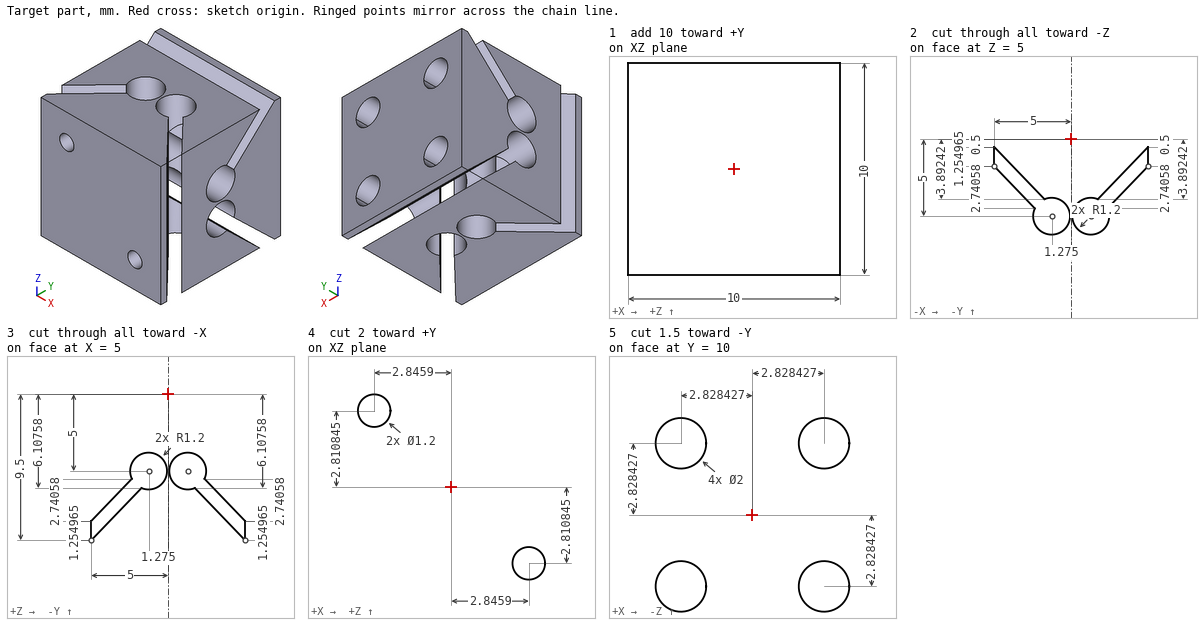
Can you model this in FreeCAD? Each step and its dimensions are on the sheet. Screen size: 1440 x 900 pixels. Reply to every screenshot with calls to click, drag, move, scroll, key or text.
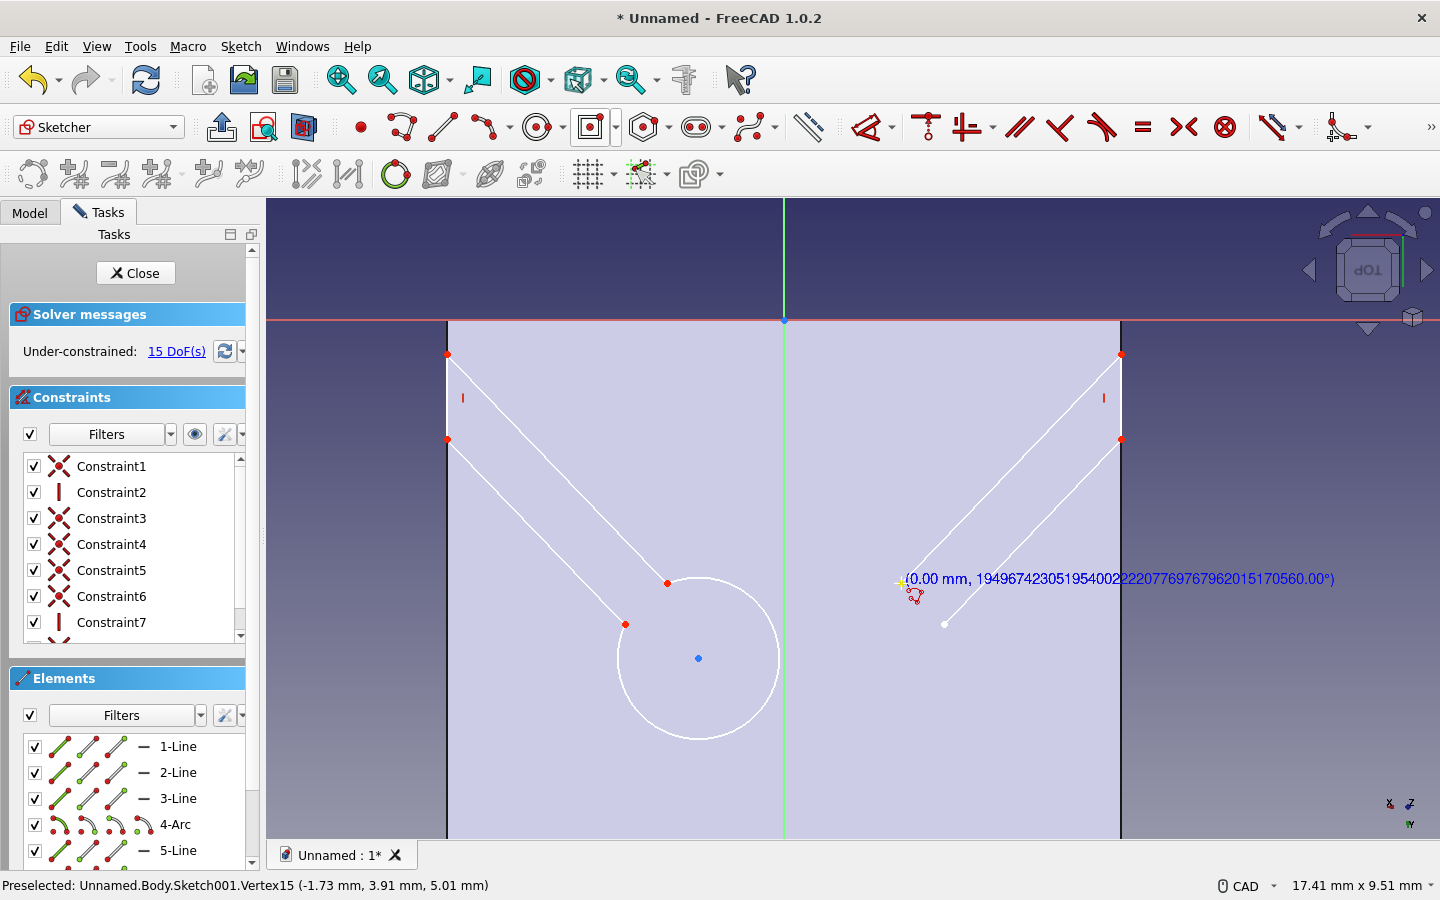
click(484, 128)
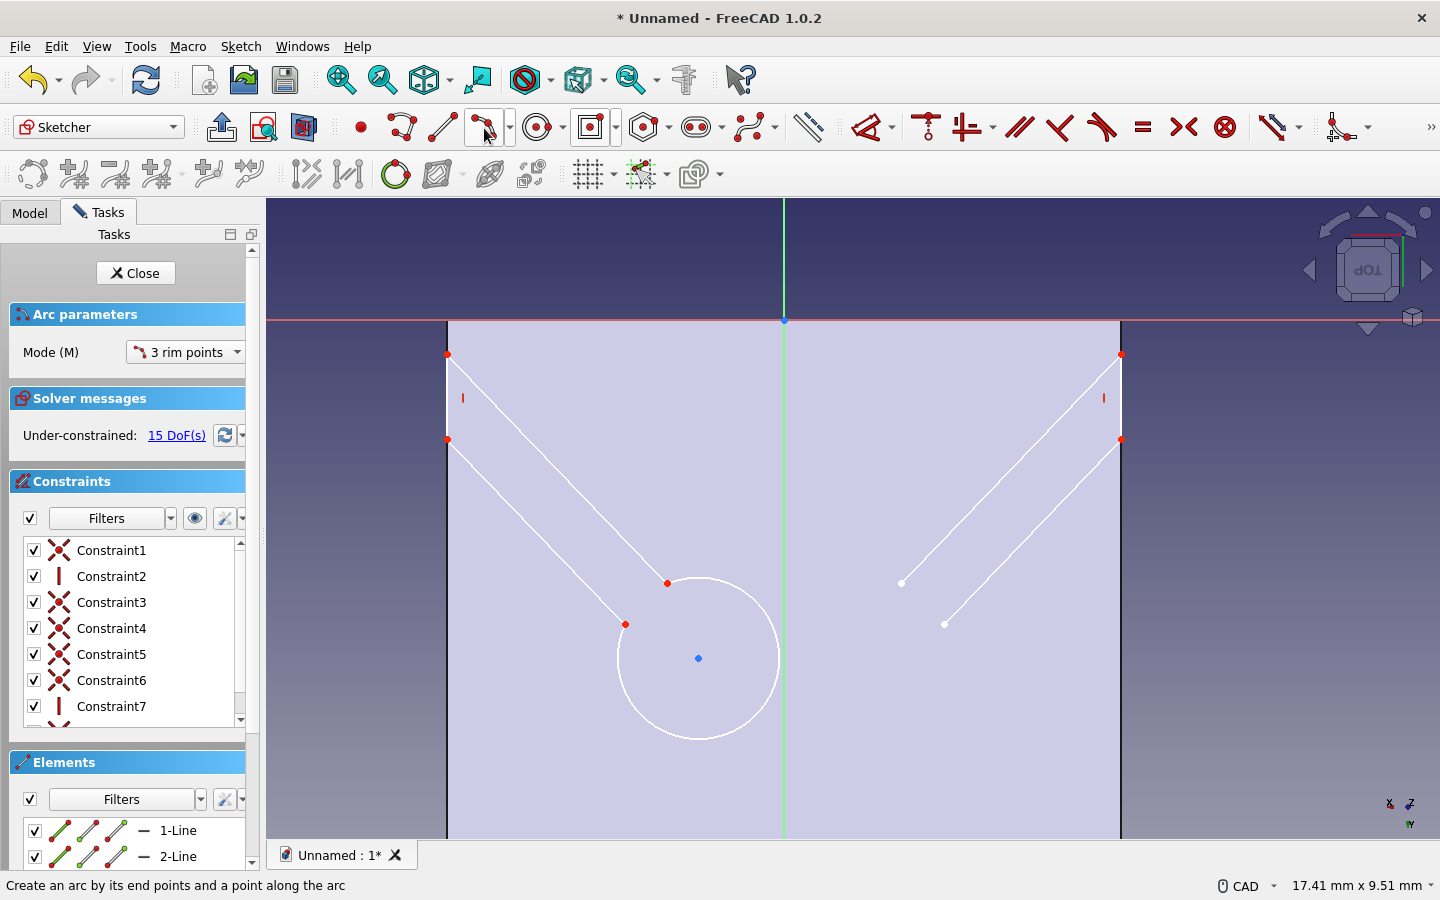
click(901, 584)
click(944, 625)
click(814, 716)
key(Escape)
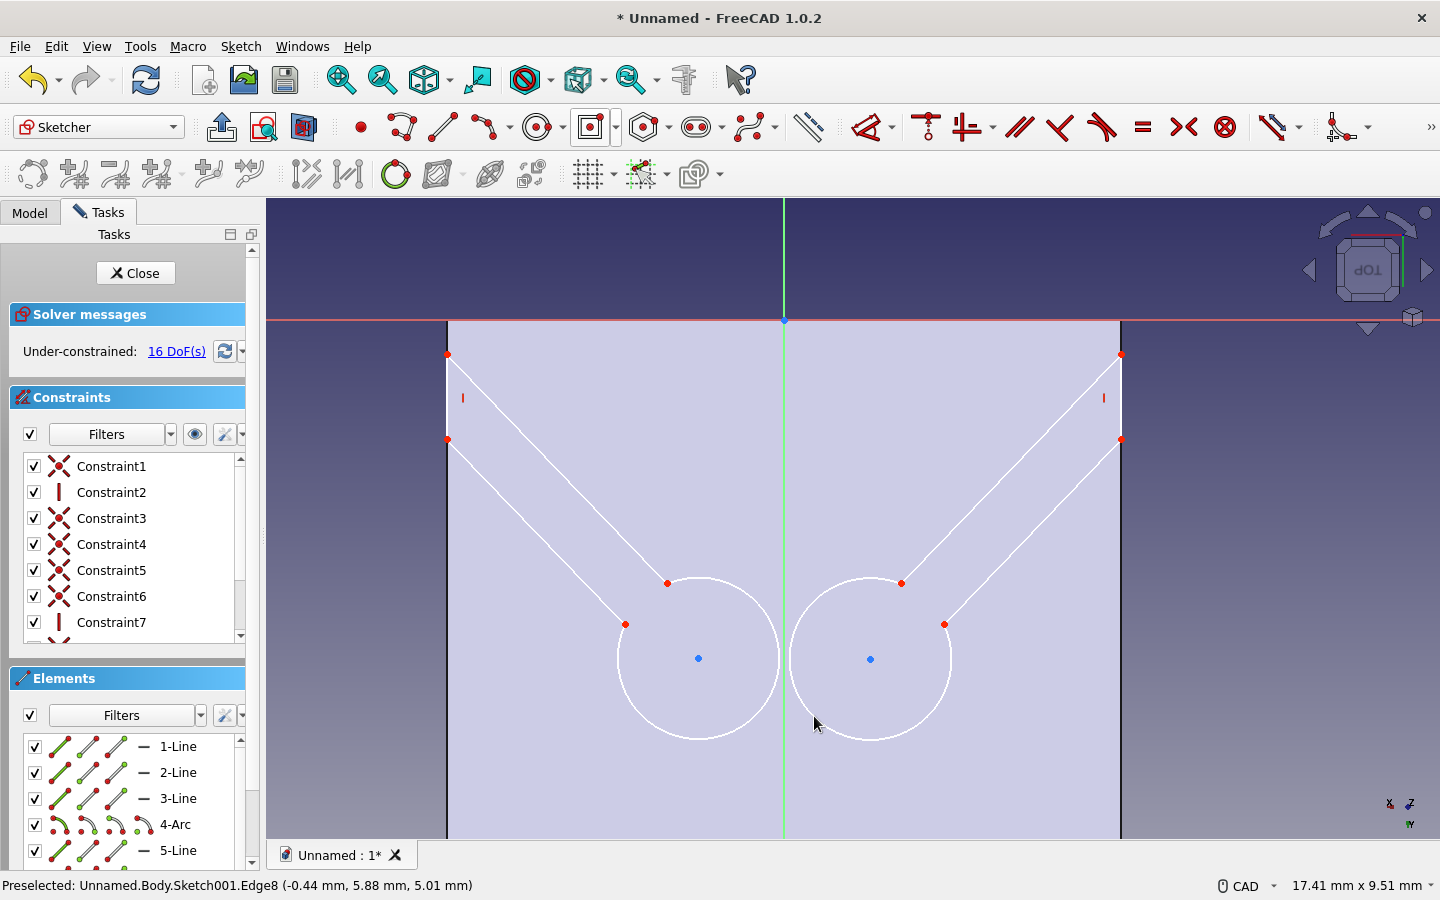
click(672, 735)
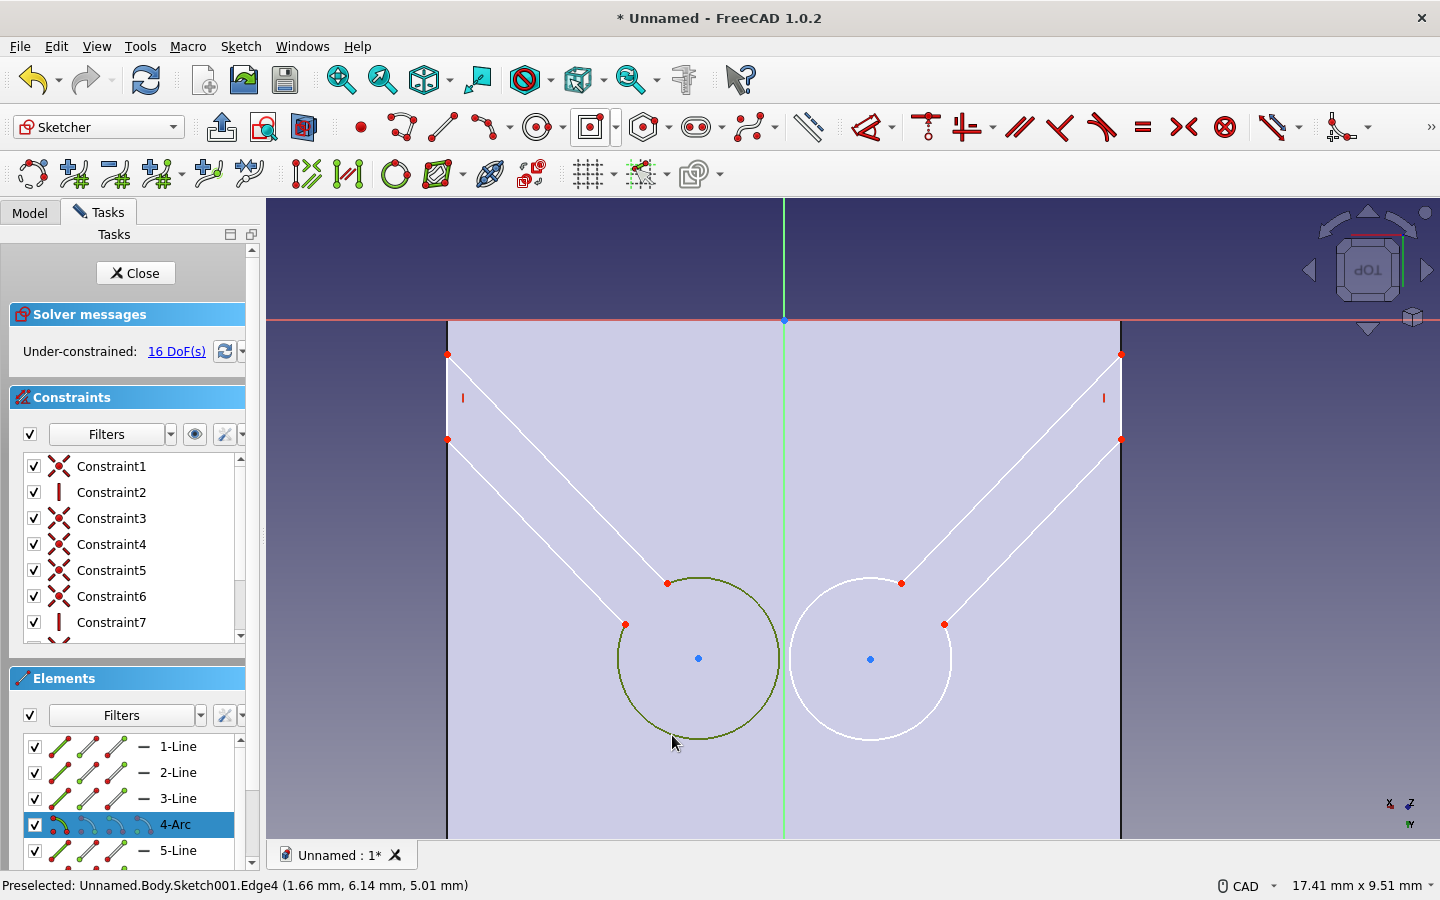
click(898, 735)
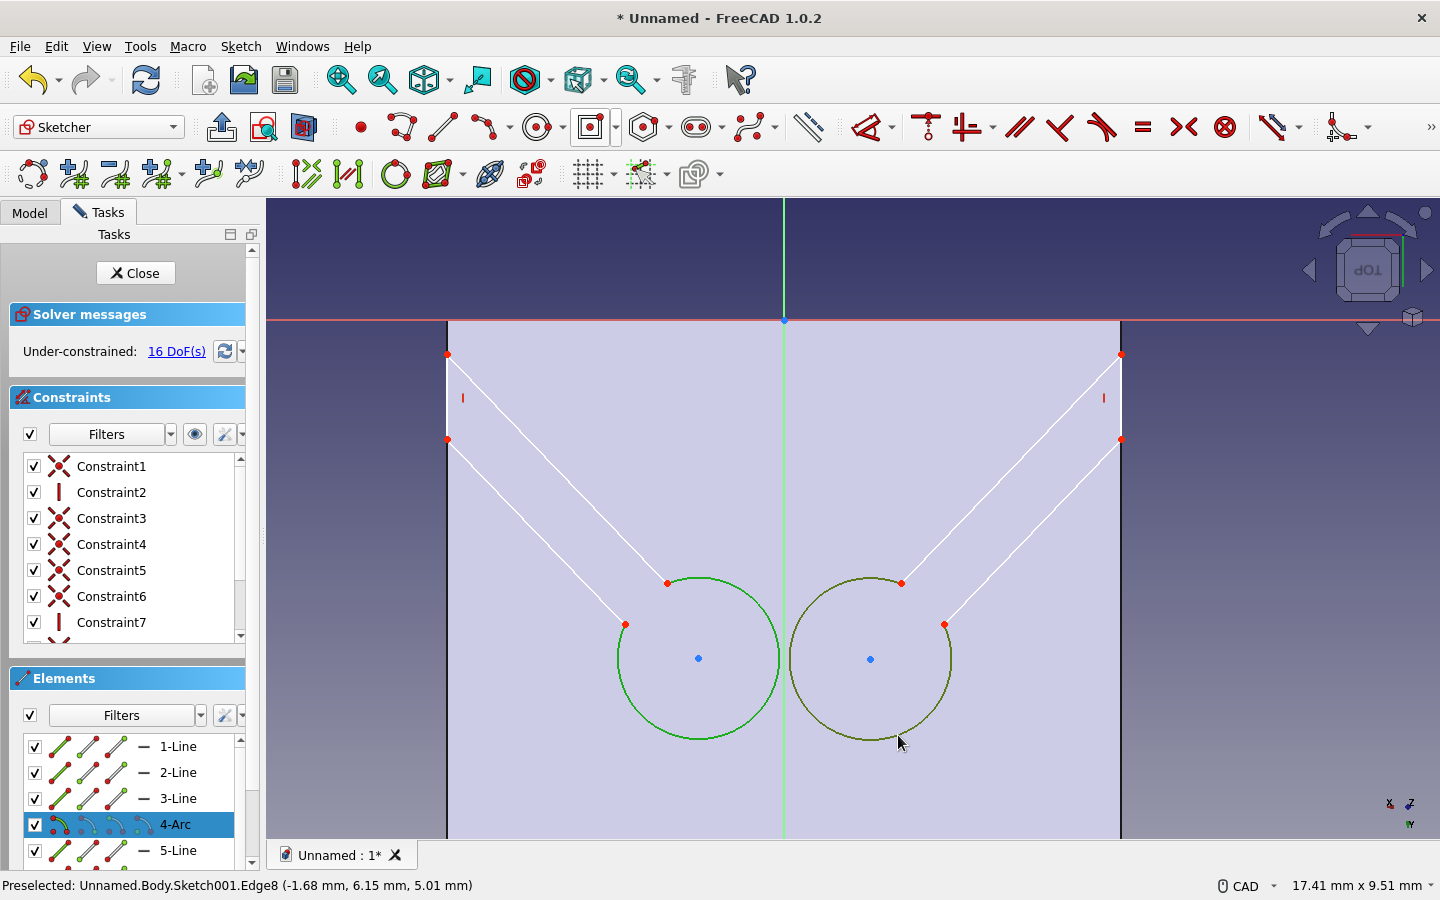
click(1143, 128)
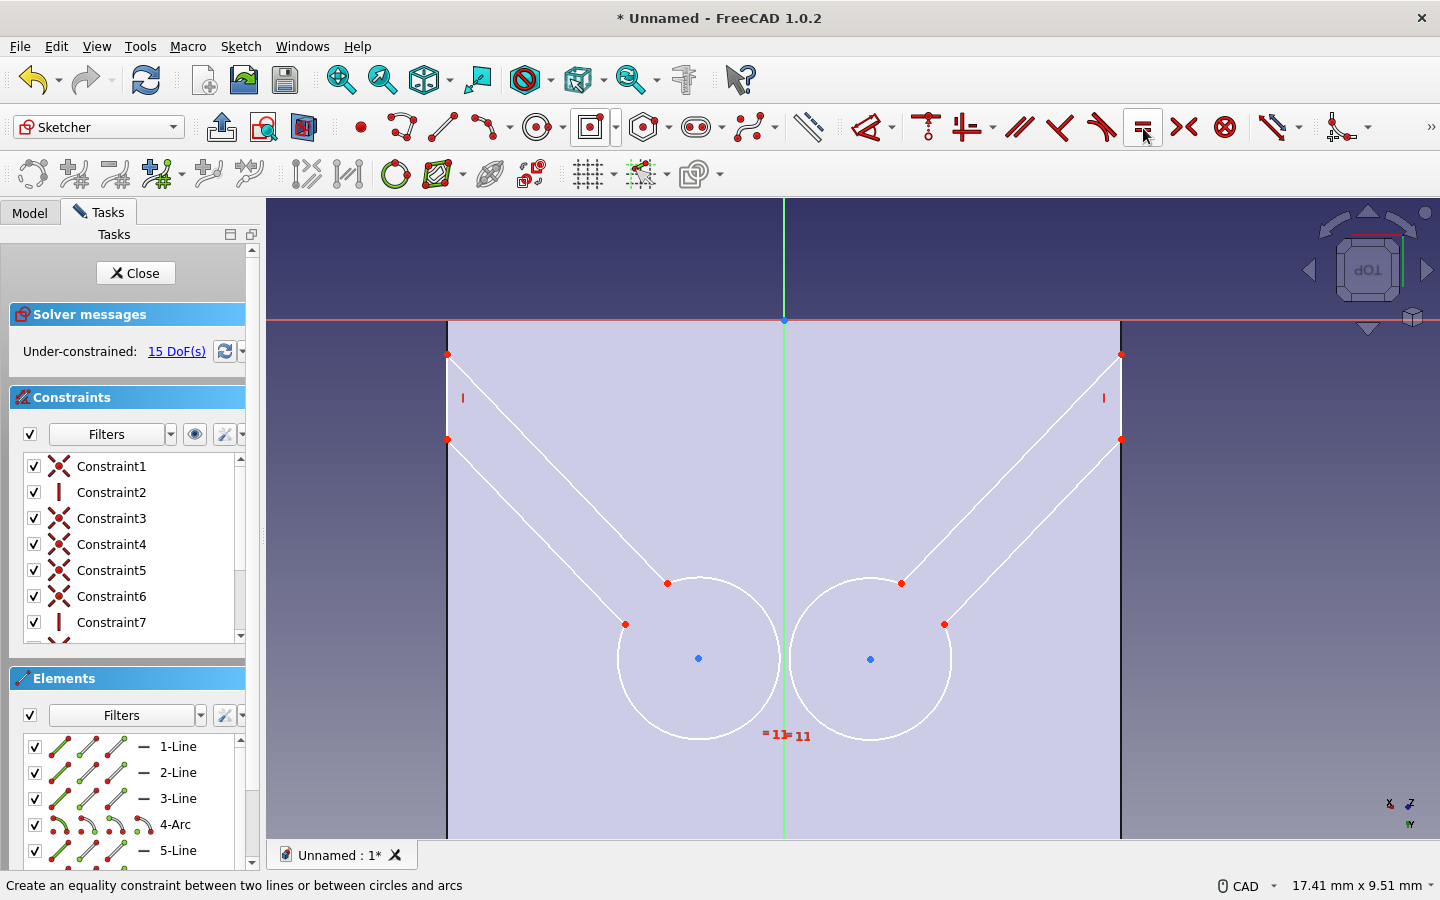
click(699, 658)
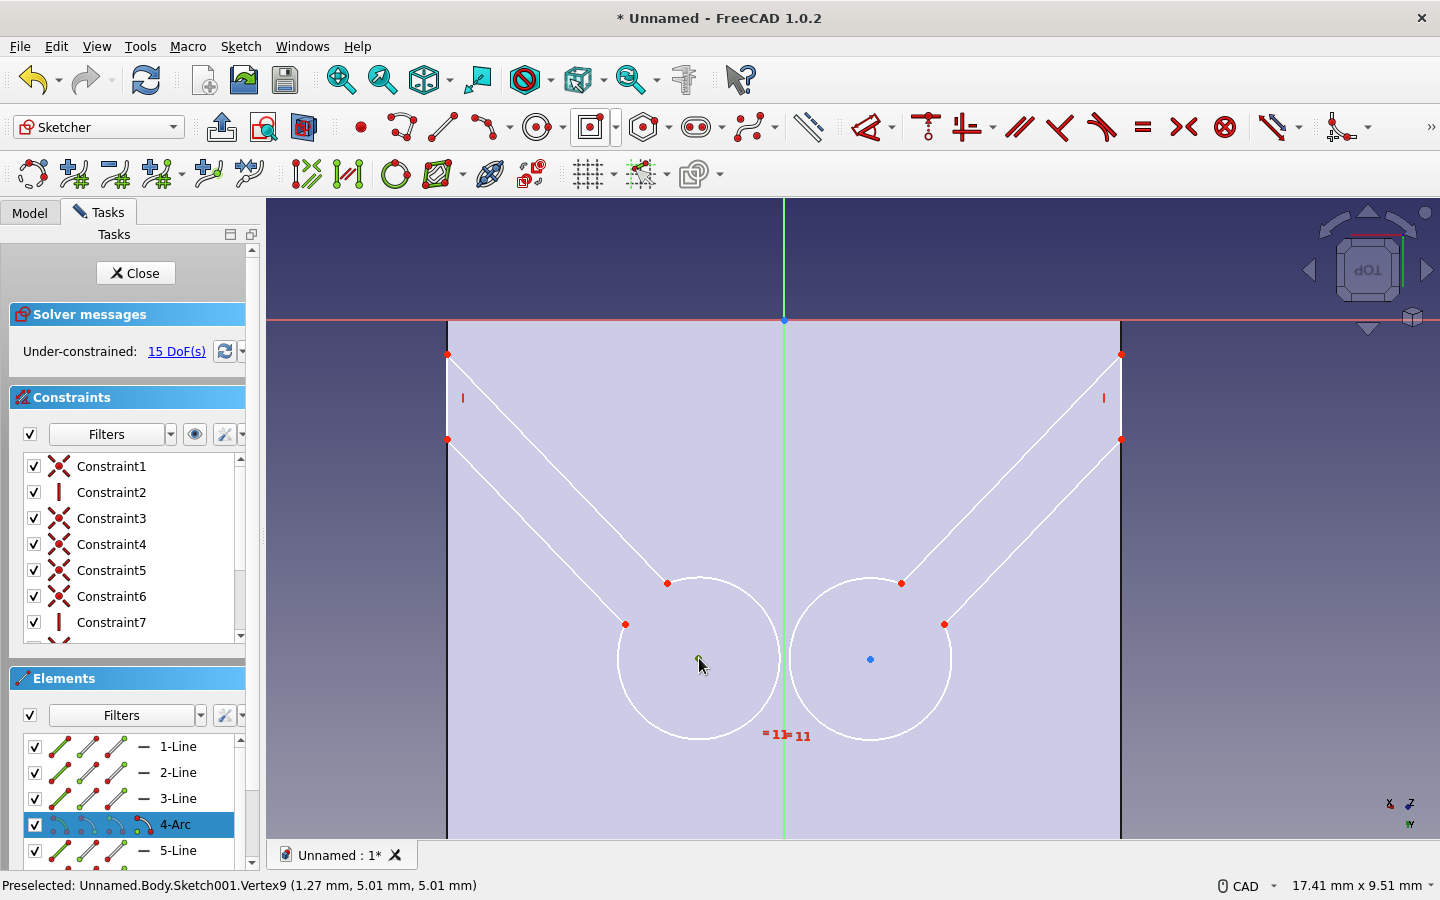
click(871, 659)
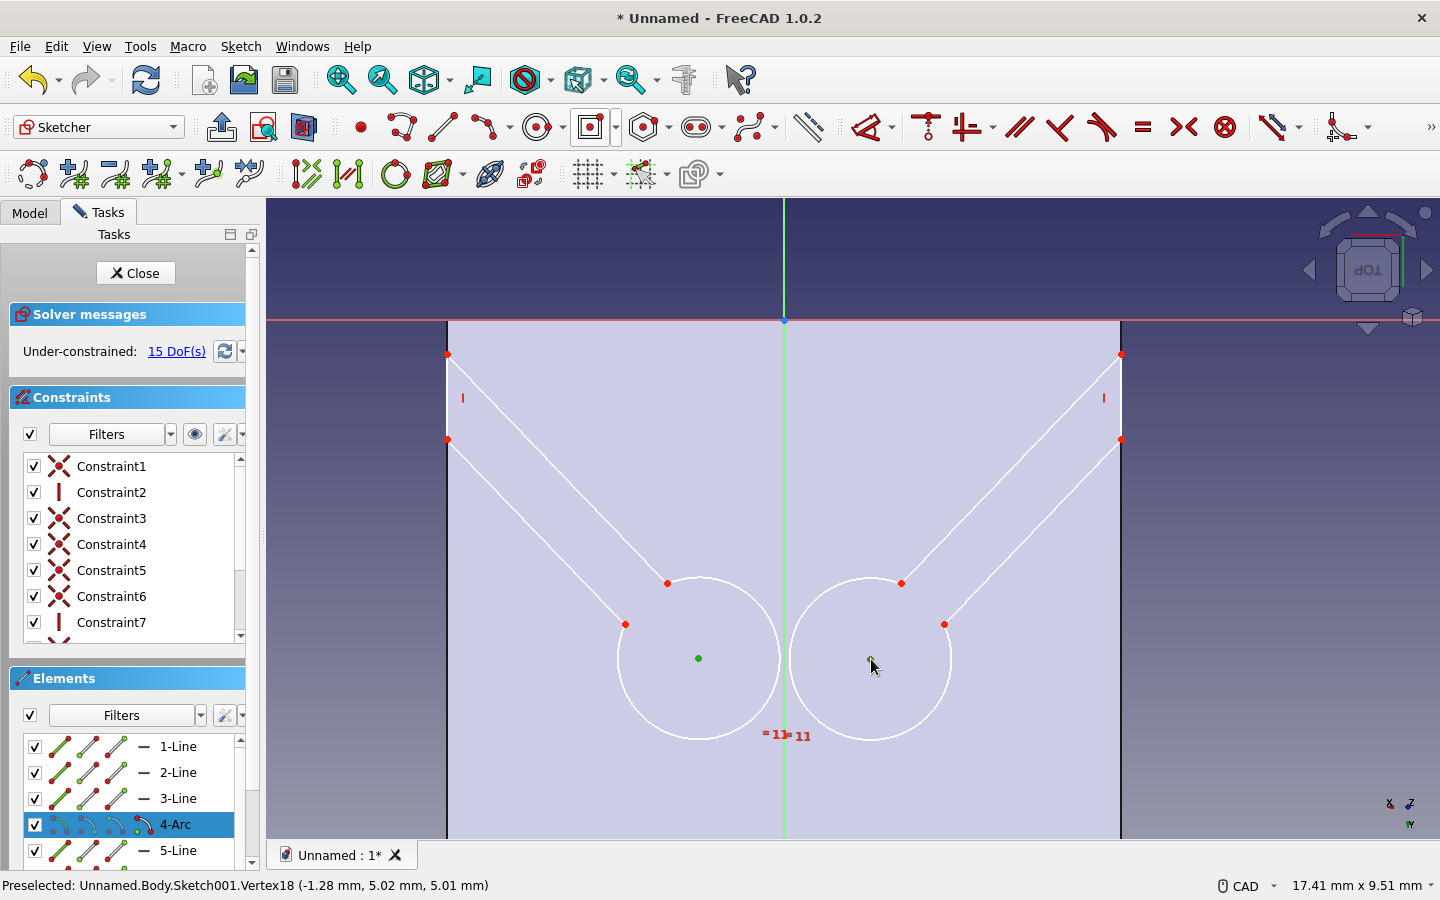
click(784, 769)